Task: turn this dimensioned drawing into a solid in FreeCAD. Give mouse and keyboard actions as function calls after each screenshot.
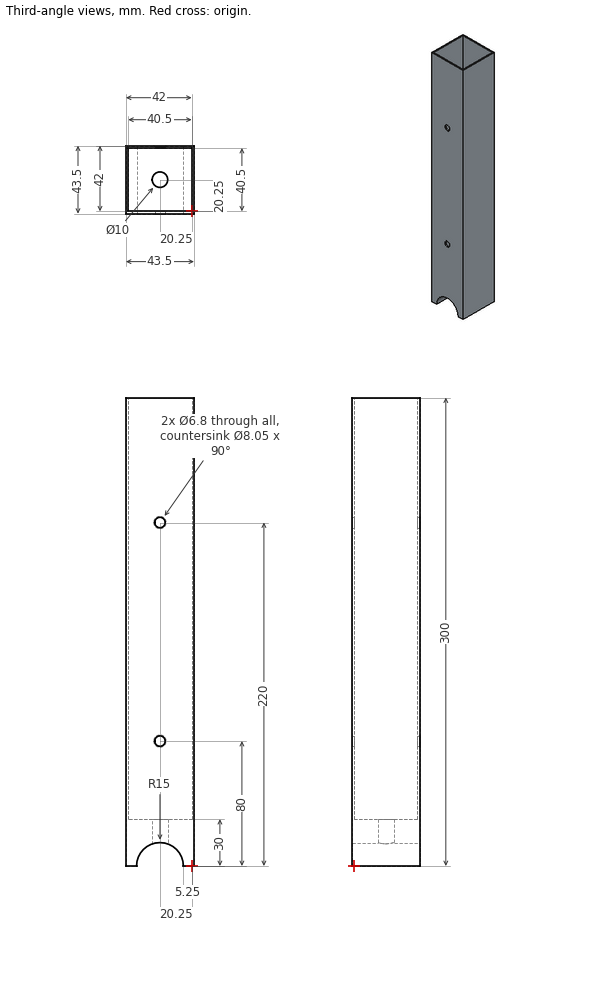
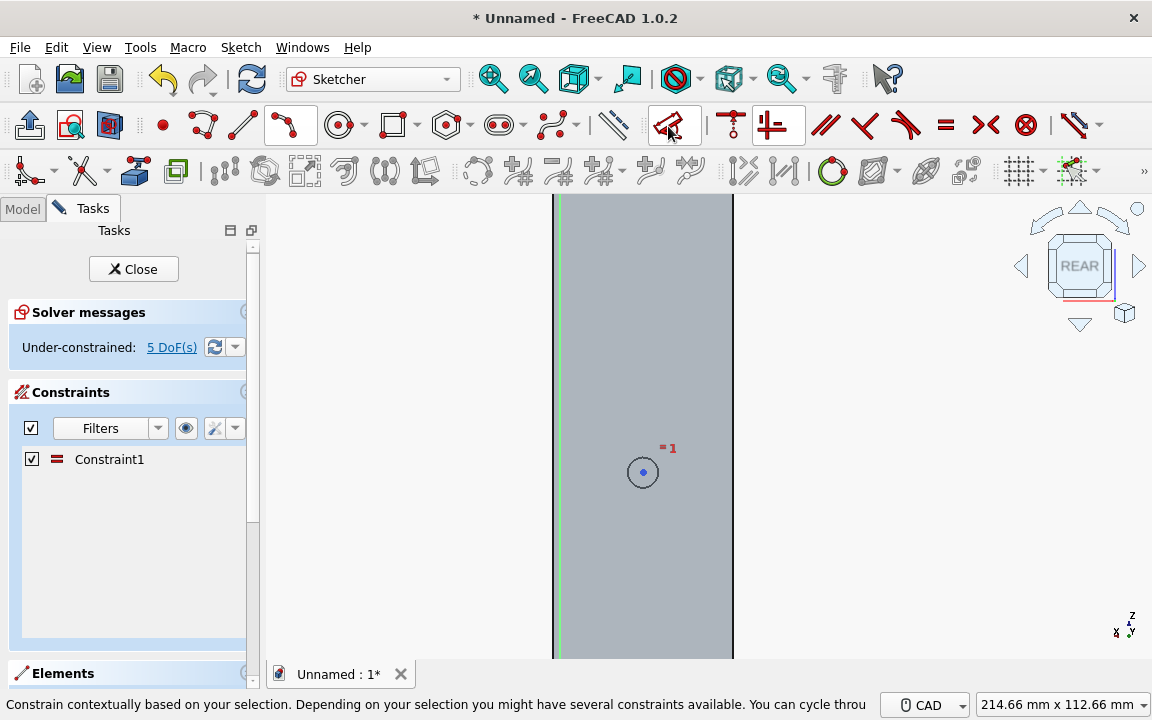
scroll(654, 464, down, 6)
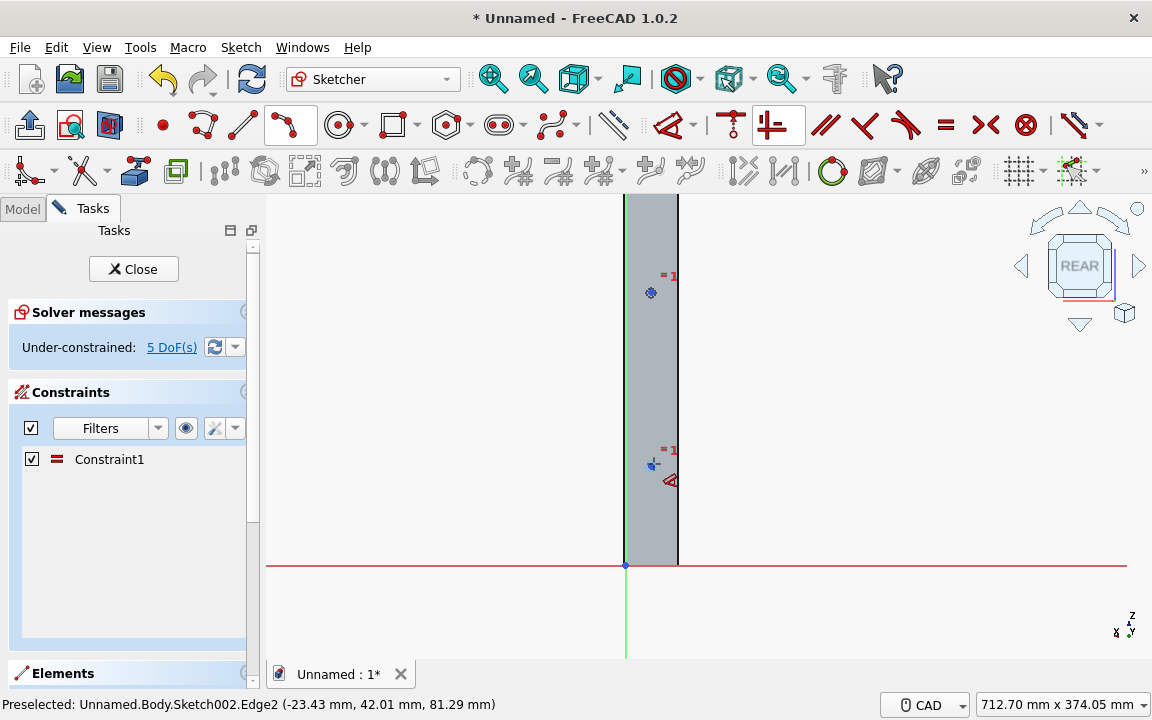
scroll(654, 290, up, 8)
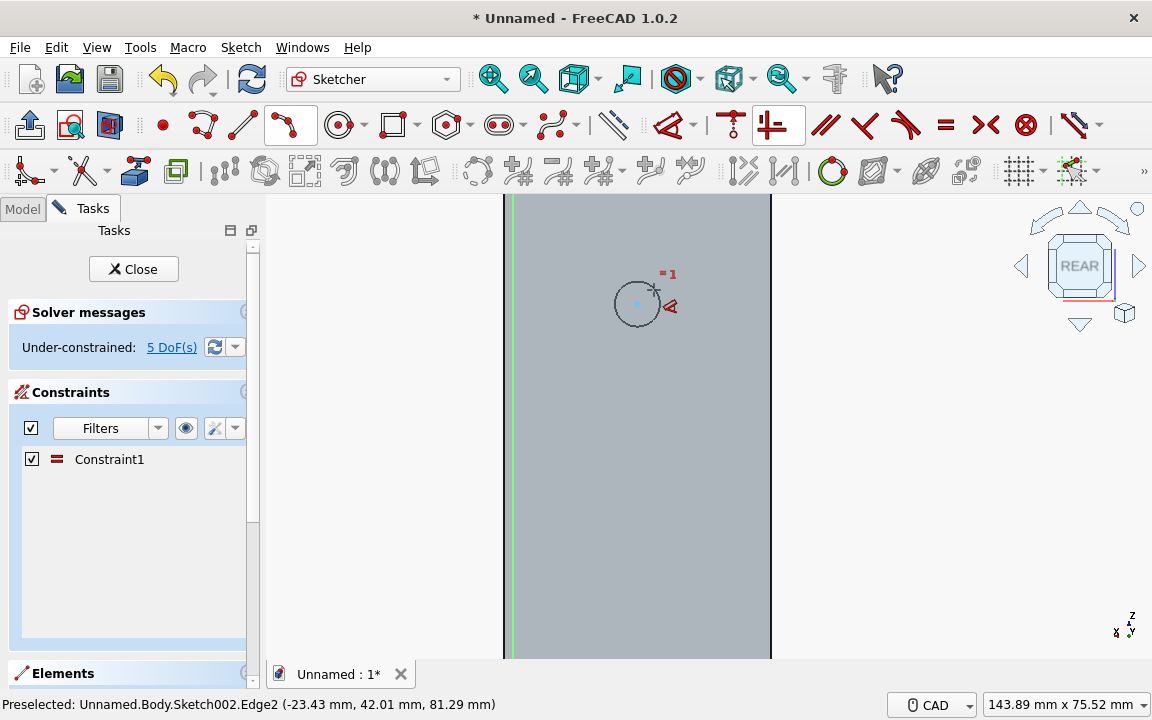
click(653, 288)
click(675, 265)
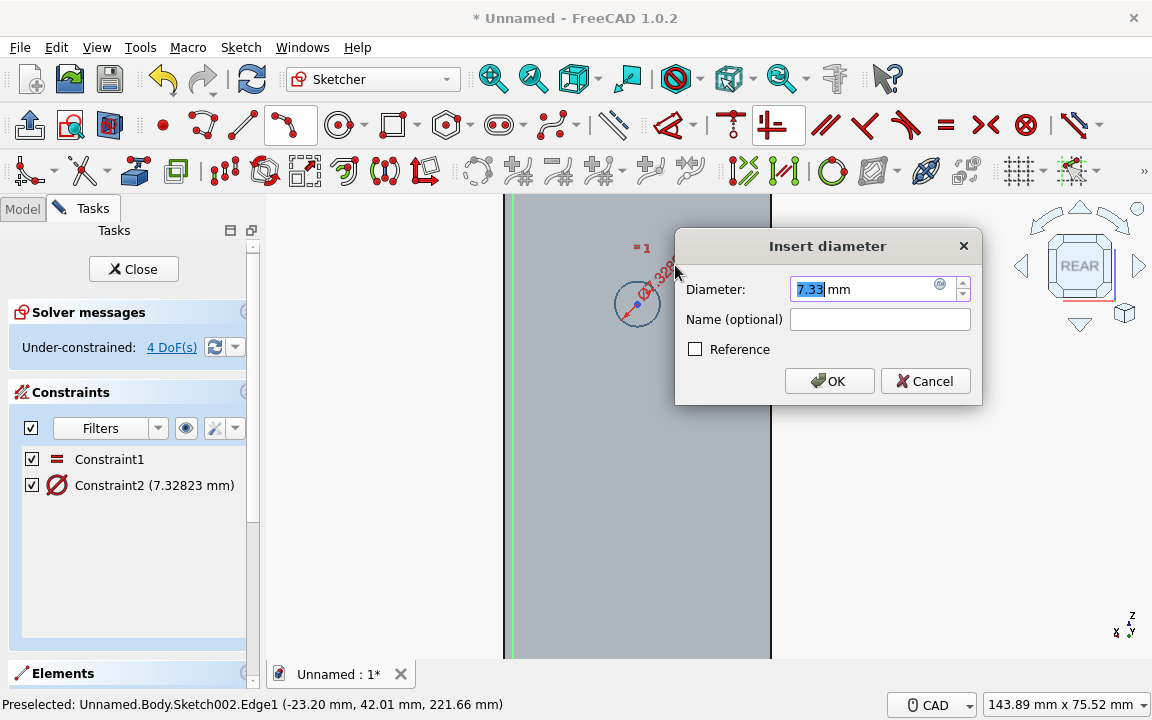
text(6.8)
key(Return)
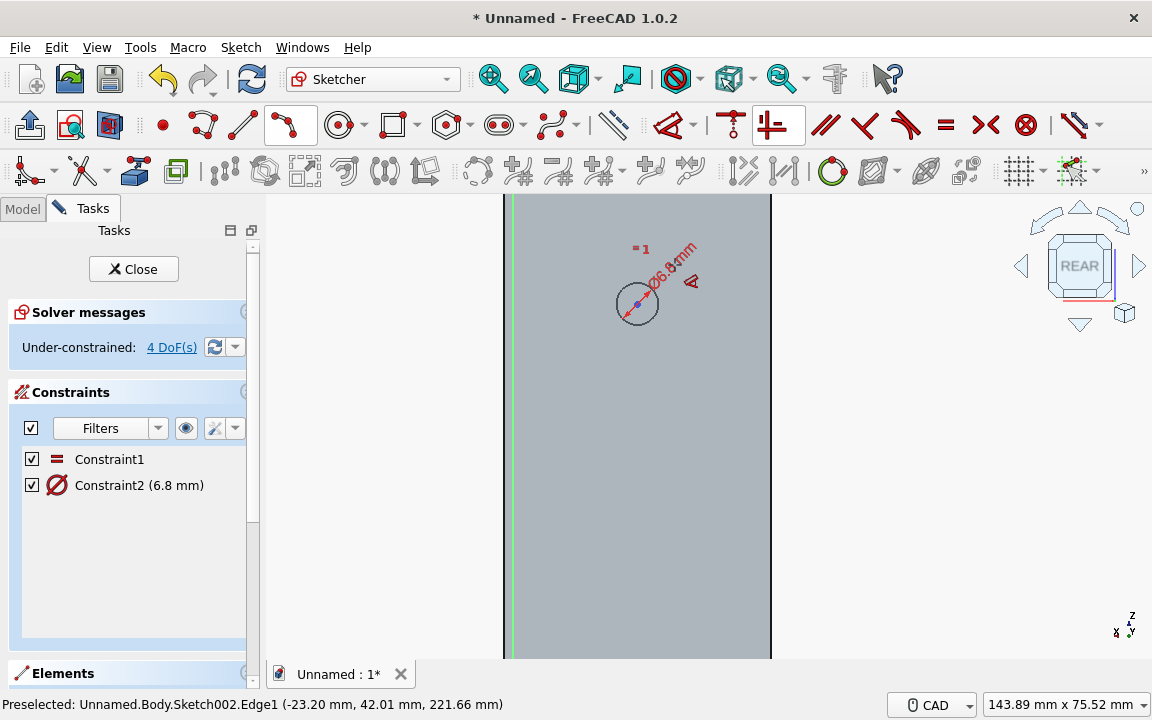
scroll(654, 290, down, 8)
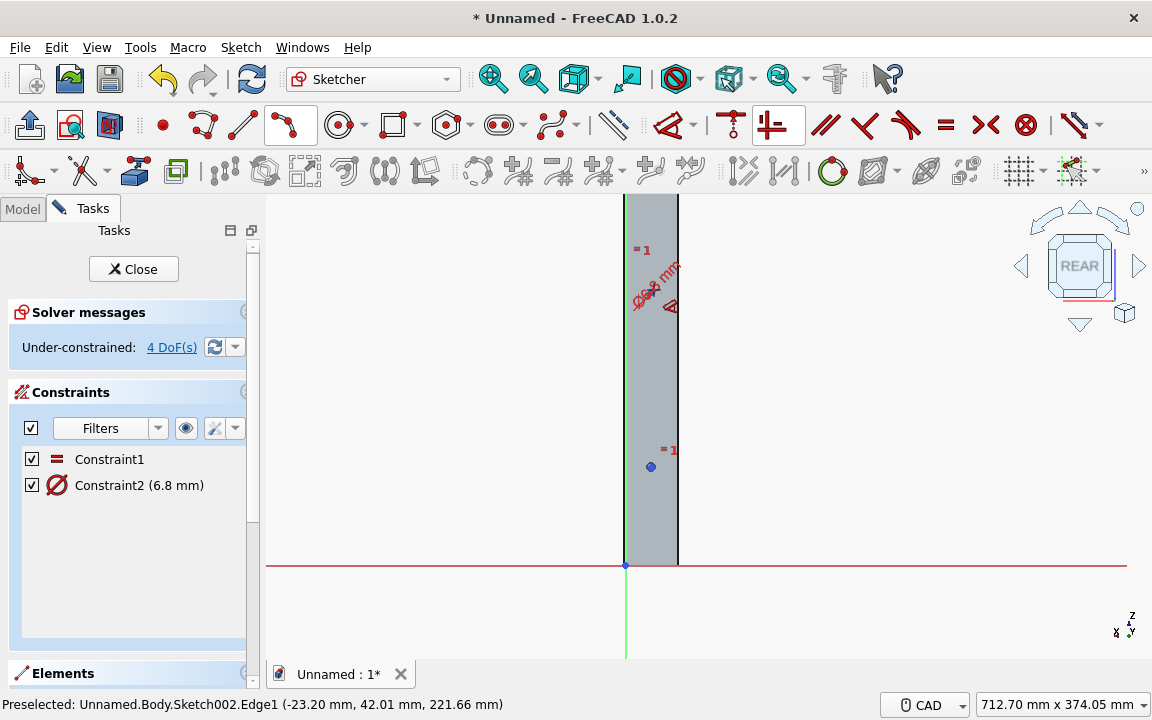
click(651, 467)
click(592, 516)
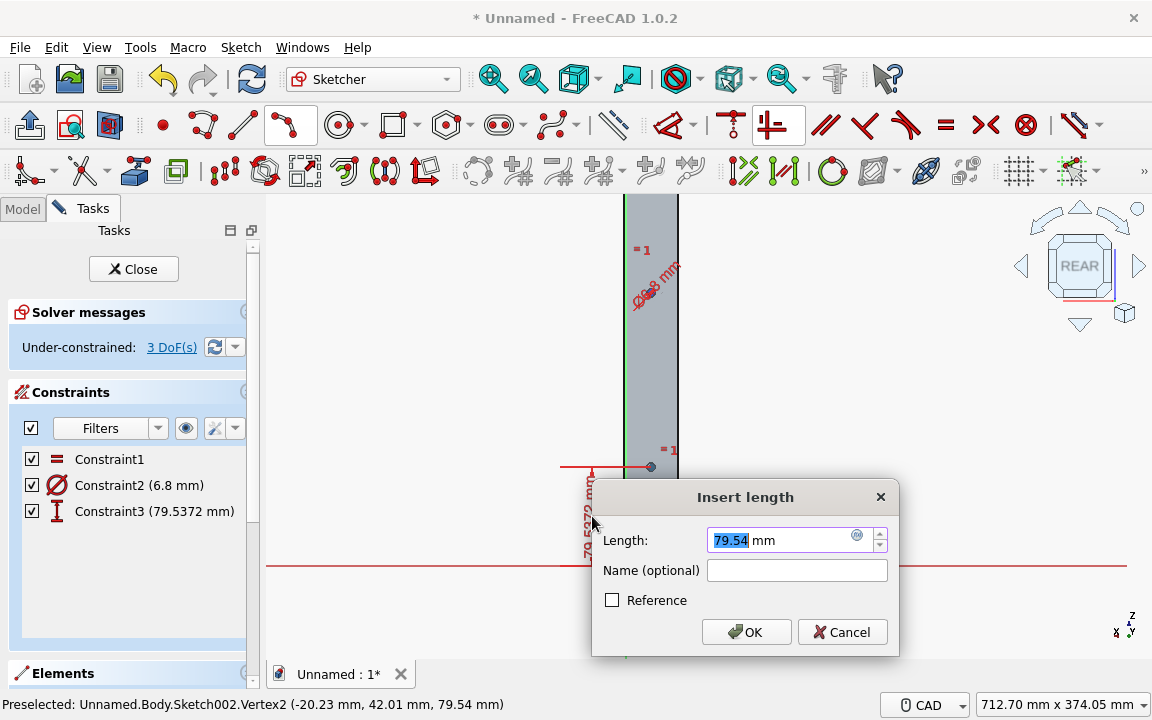
text(80)
key(Return)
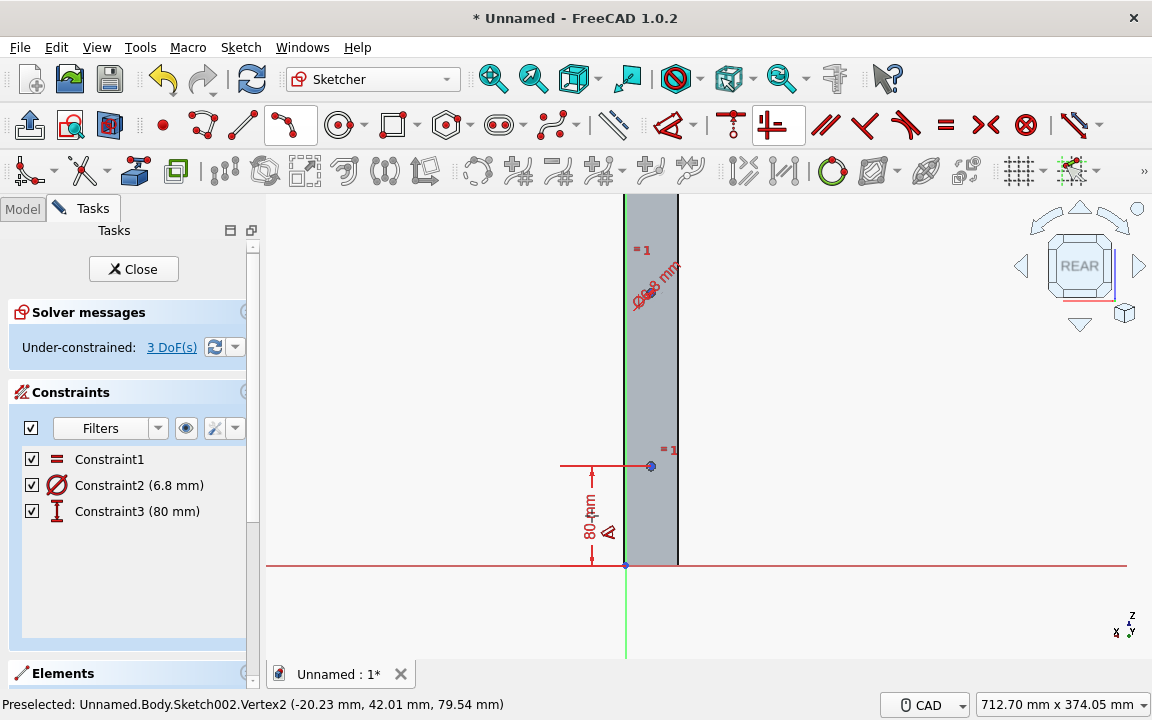
click(651, 293)
click(592, 429)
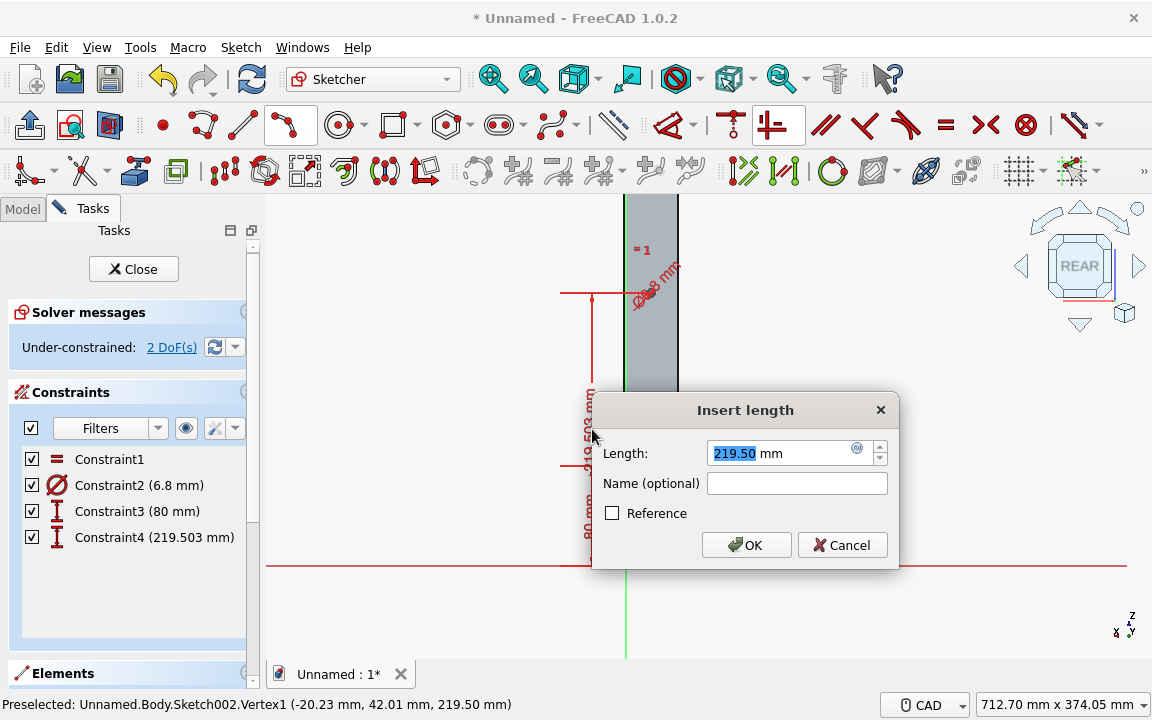
text(220)
key(Return)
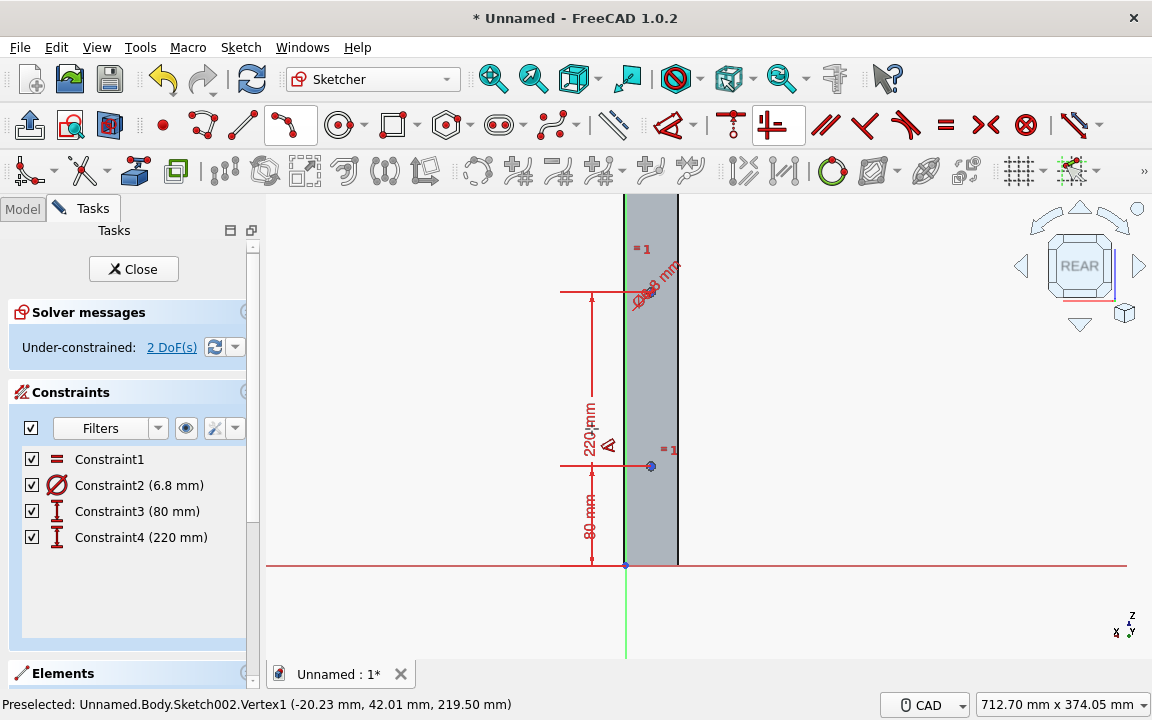
scroll(651, 292, up, 3)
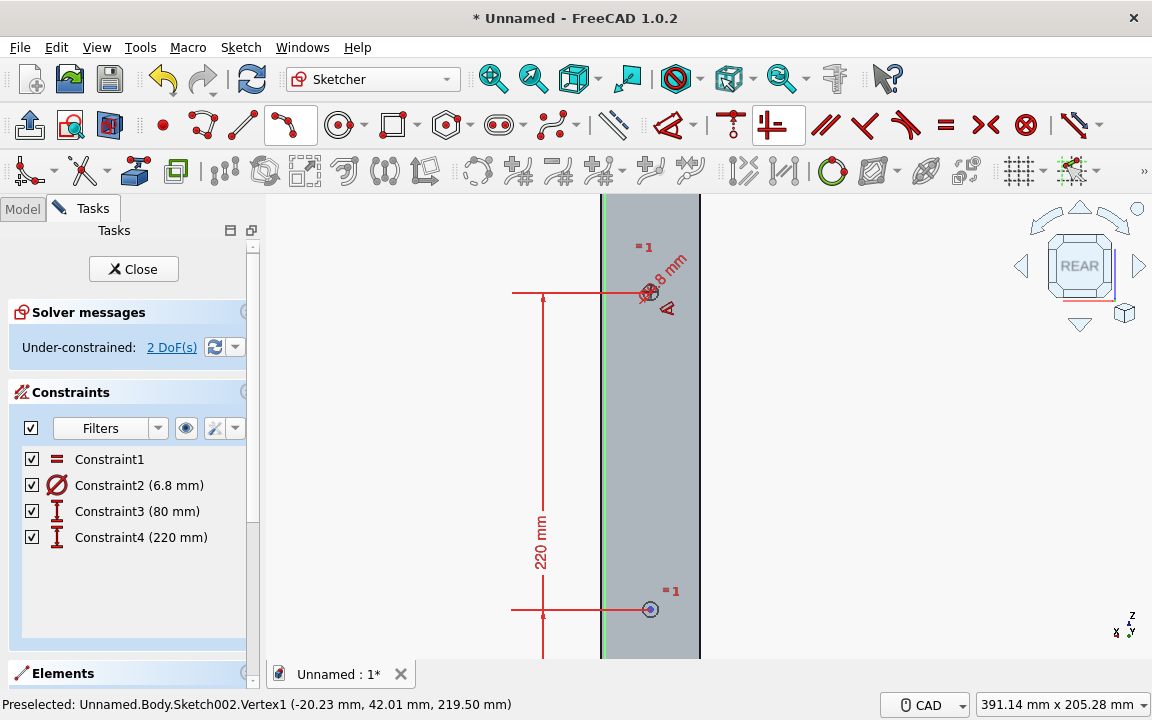
click(651, 293)
click(628, 259)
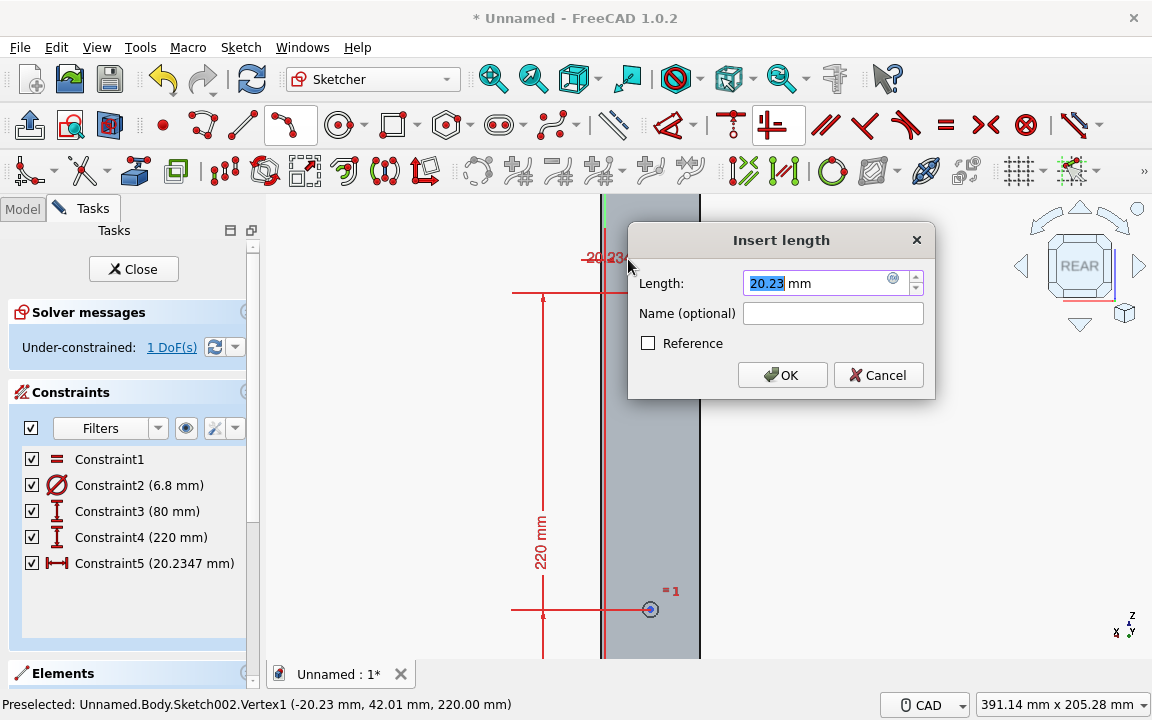
text(20.25)
key(Return)